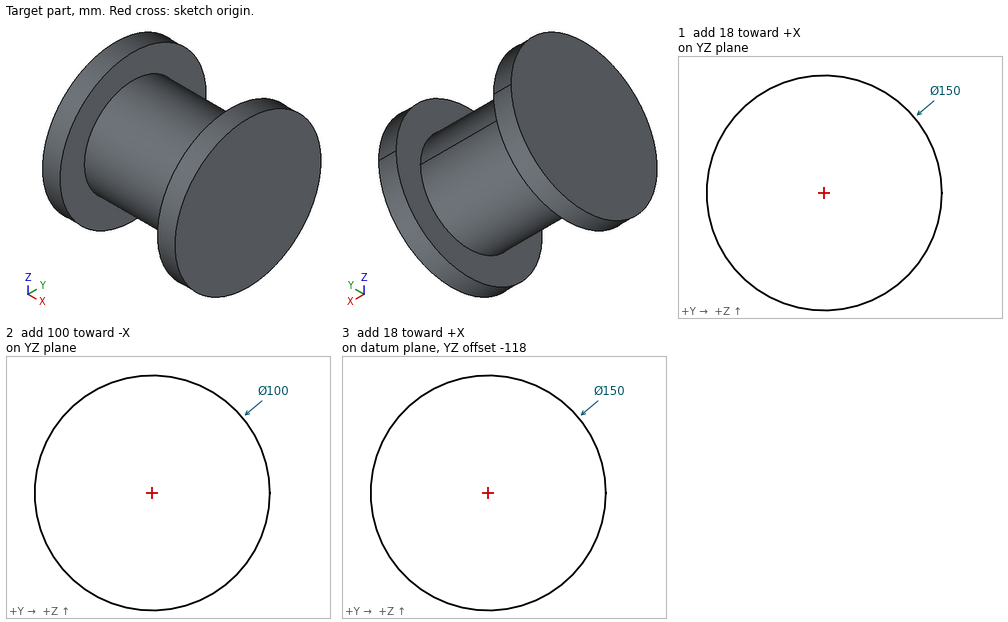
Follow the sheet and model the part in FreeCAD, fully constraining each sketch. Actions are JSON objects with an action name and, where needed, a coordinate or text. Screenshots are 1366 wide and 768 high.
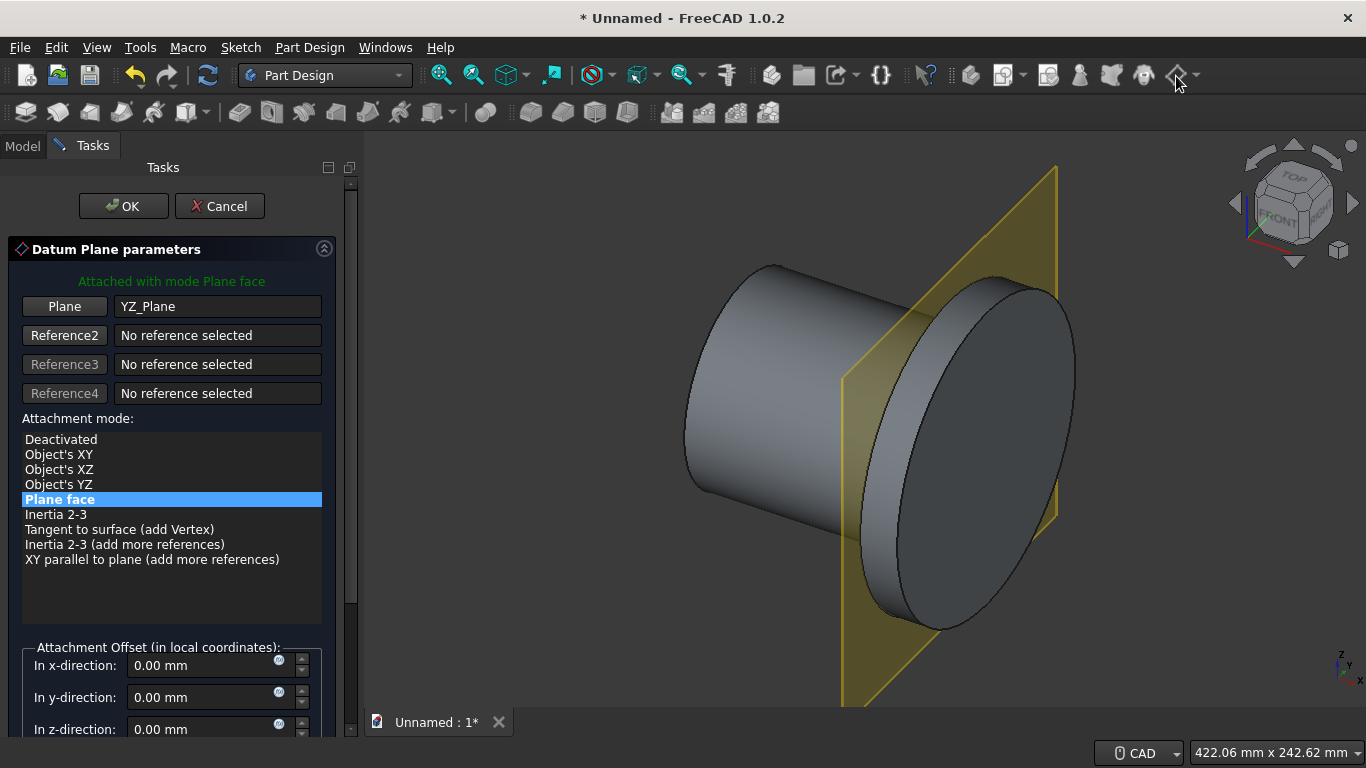
{"action": "scroll", "coordinate": [351, 456], "scroll_direction": "down", "scroll_amount": 2}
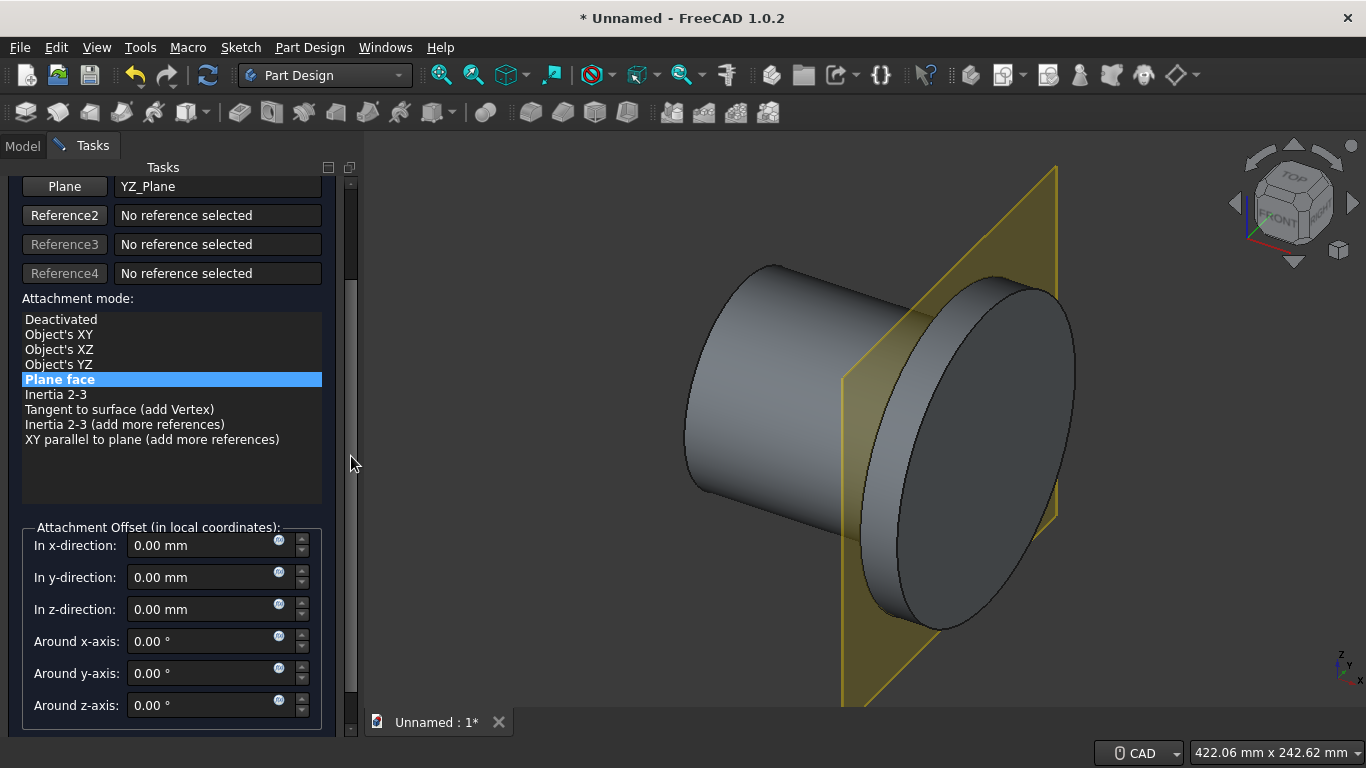
{"action": "triple_click", "coordinate": [210, 609]}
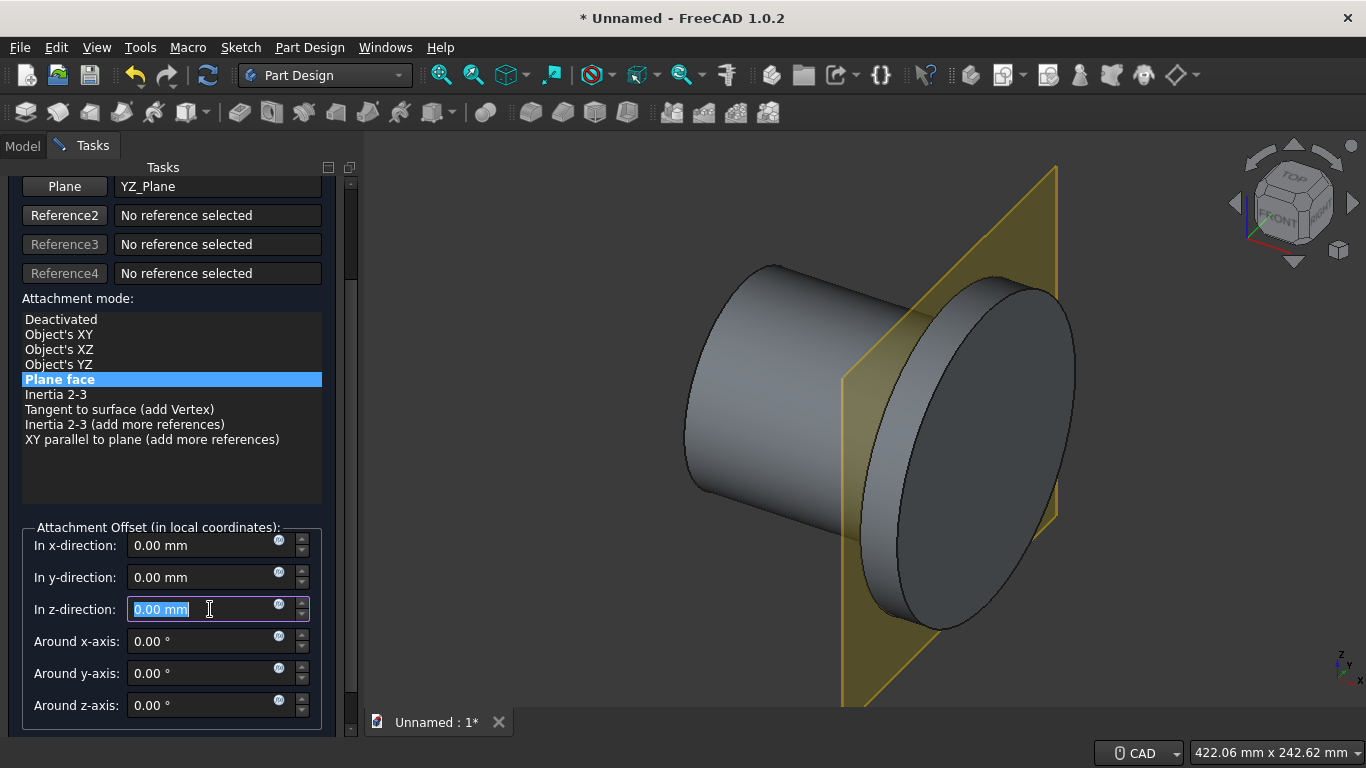
{"action": "type", "text": "-118"}
{"action": "key", "text": "Tab"}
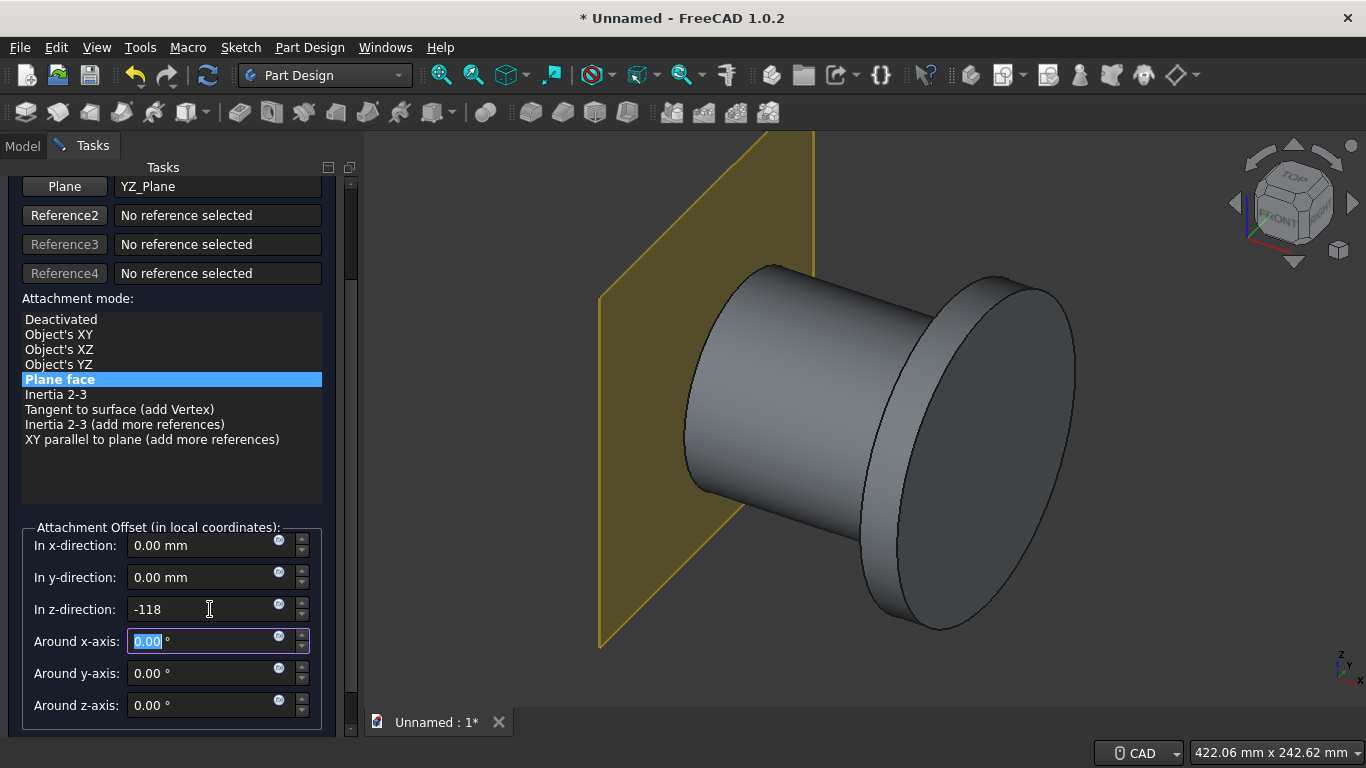
{"action": "scroll", "coordinate": [351, 456], "scroll_direction": "up", "scroll_amount": 3}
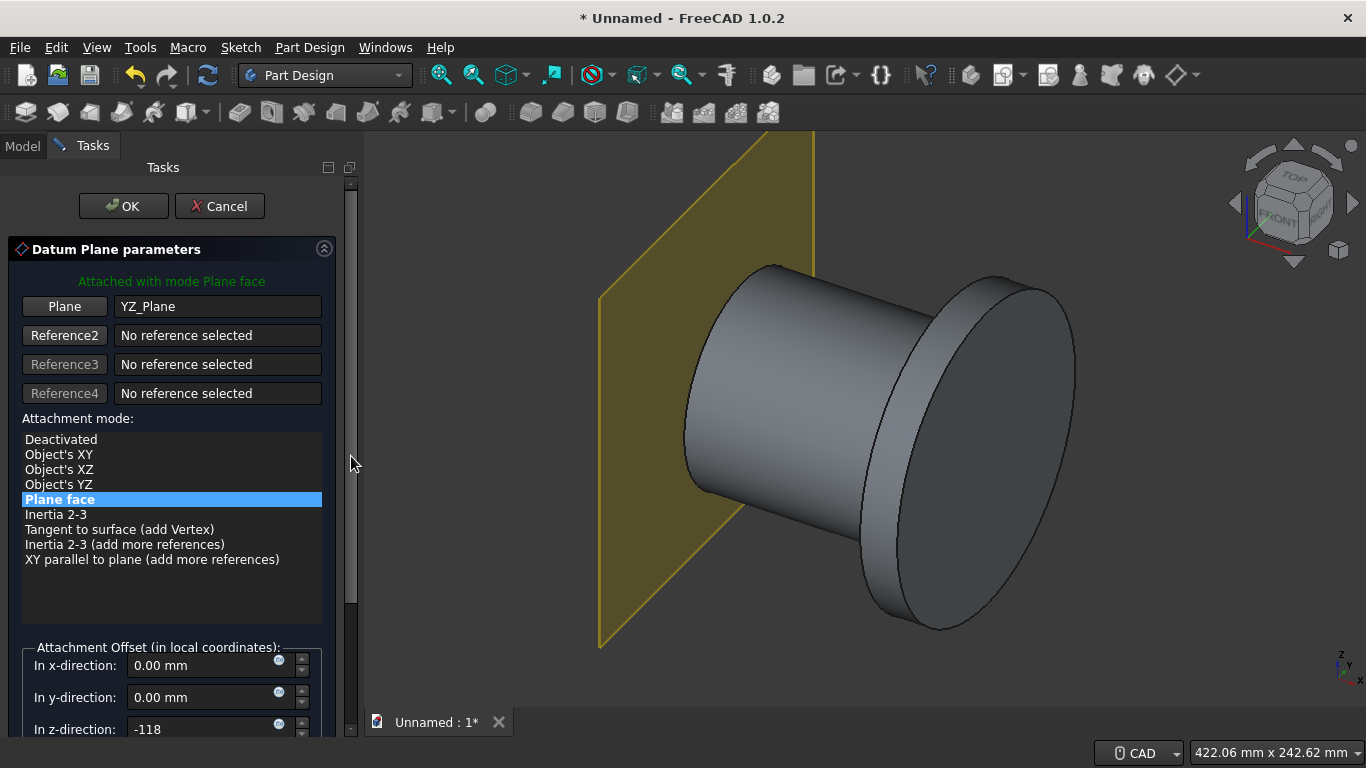
{"action": "left_click", "coordinate": [124, 206]}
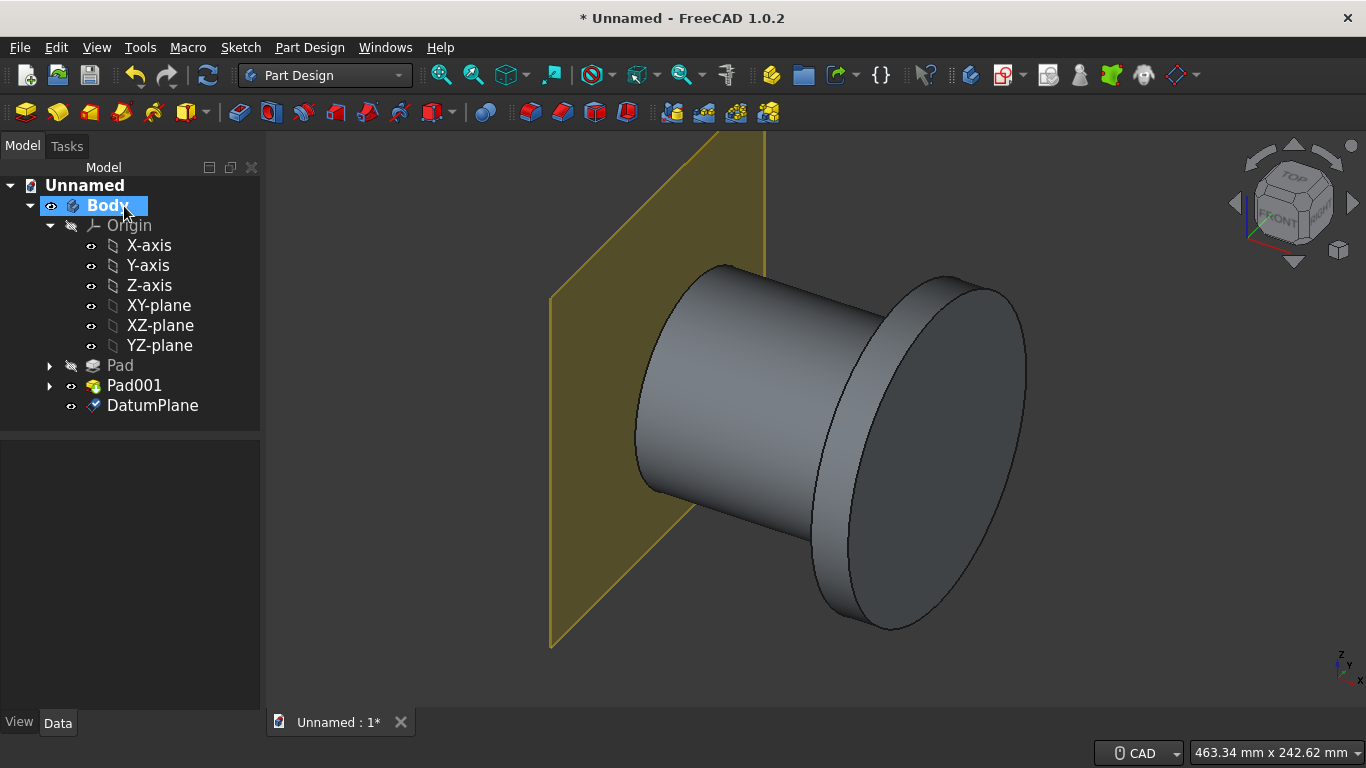
{"action": "left_click", "coordinate": [116, 406]}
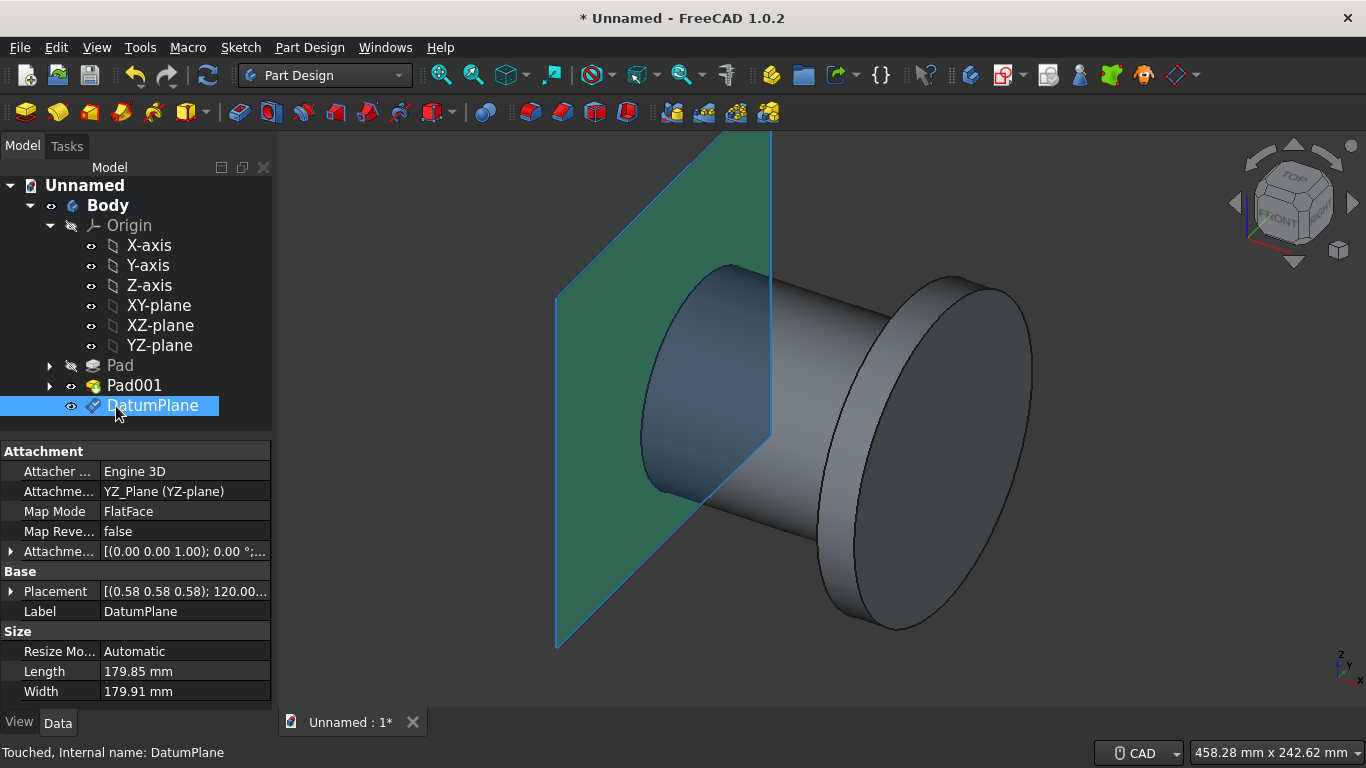
{"action": "left_click", "coordinate": [1004, 76]}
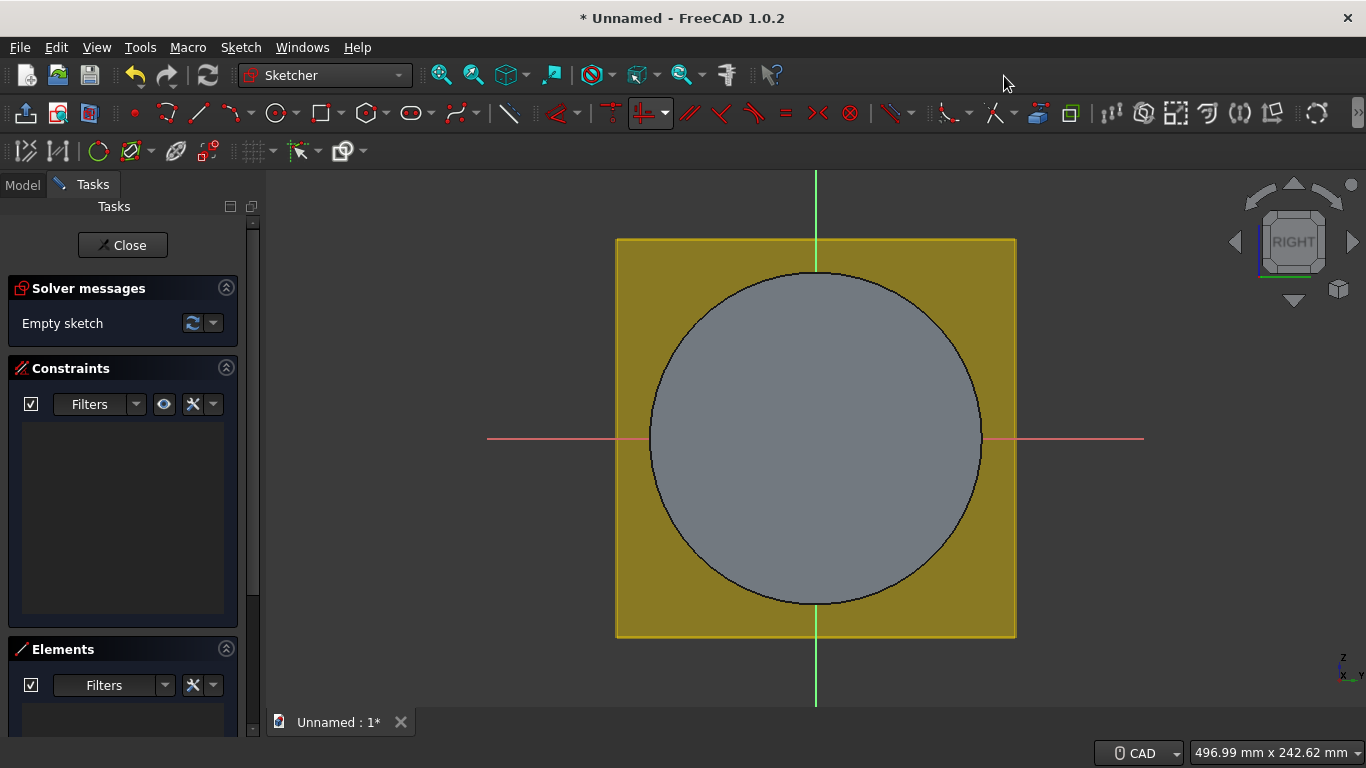
{"action": "left_click", "coordinate": [90, 114]}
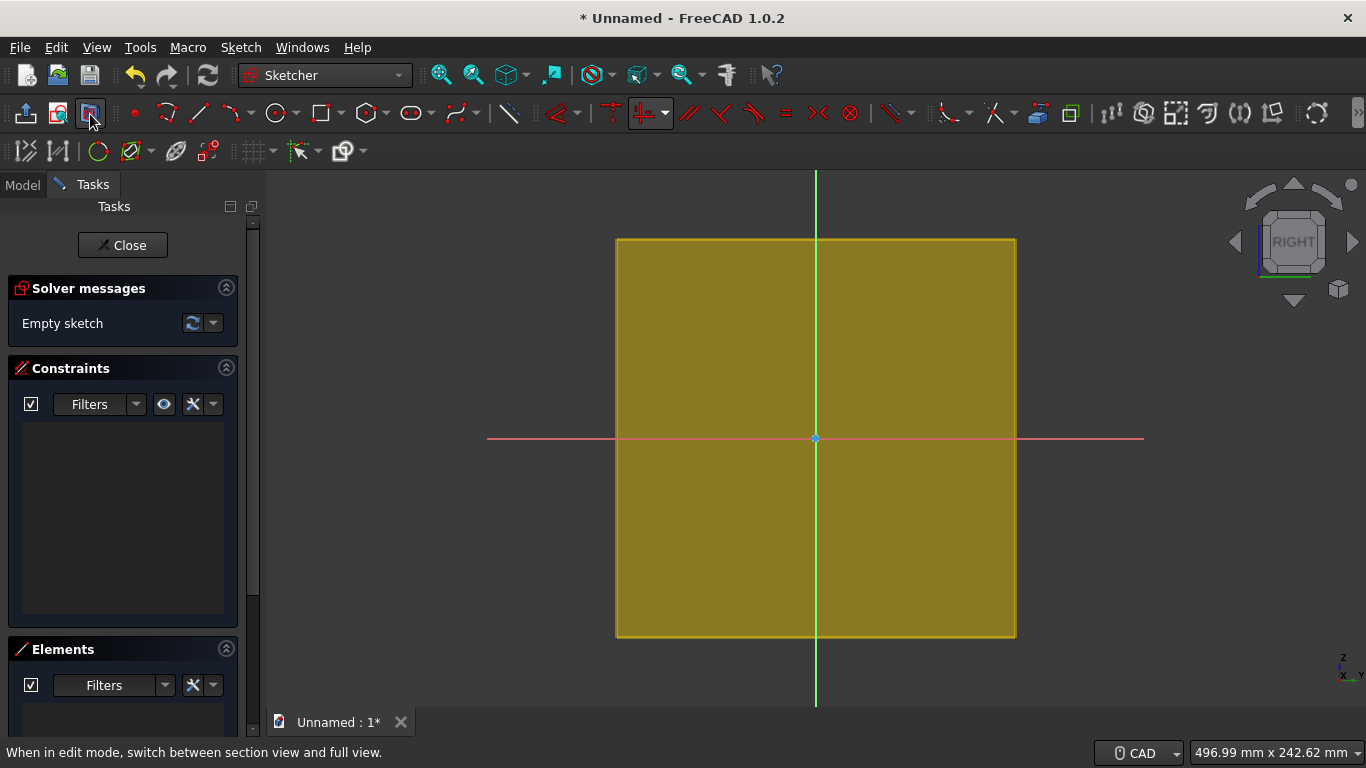
{"action": "left_click", "coordinate": [276, 114]}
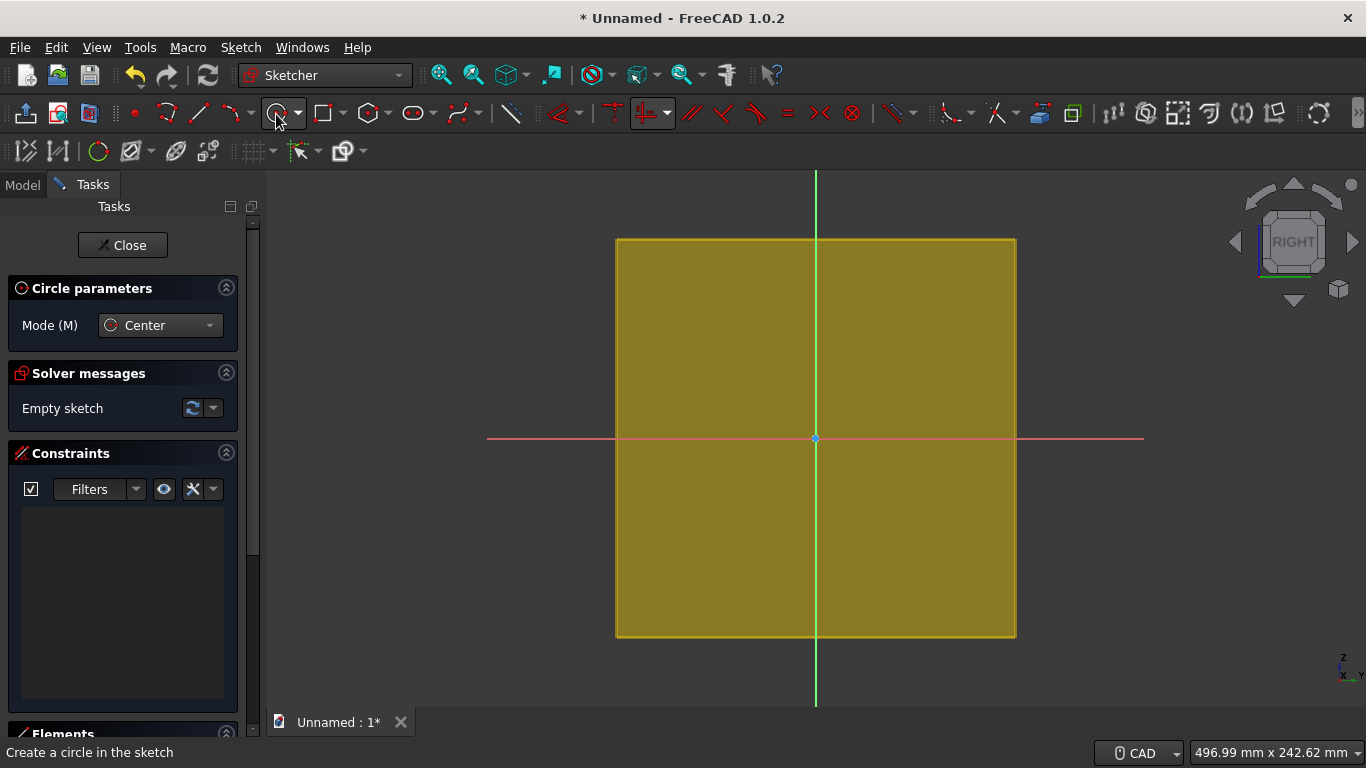
{"action": "left_click", "coordinate": [816, 438]}
{"action": "mouse_move", "coordinate": [933, 321]}